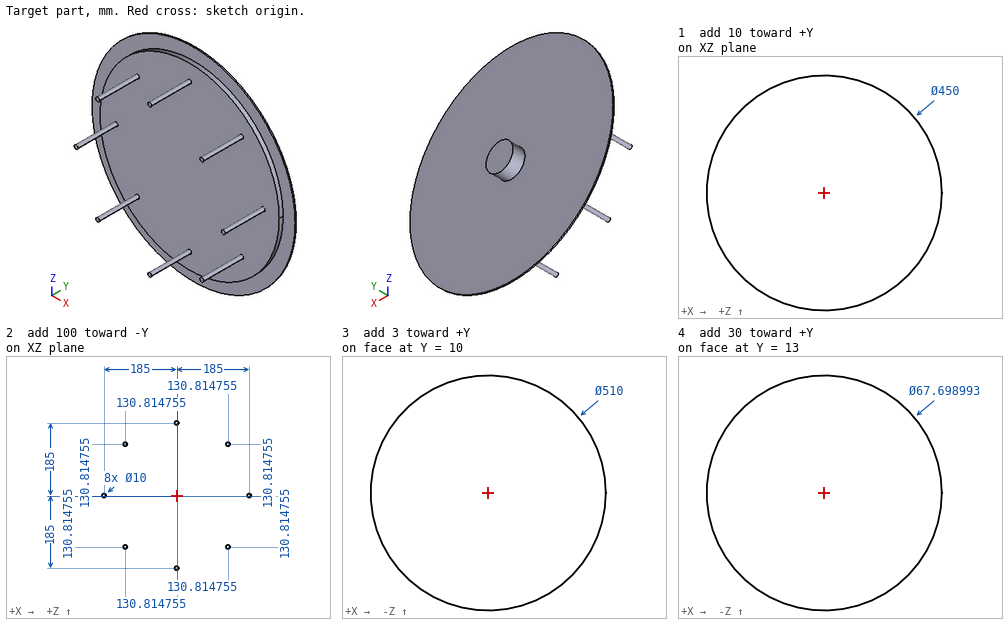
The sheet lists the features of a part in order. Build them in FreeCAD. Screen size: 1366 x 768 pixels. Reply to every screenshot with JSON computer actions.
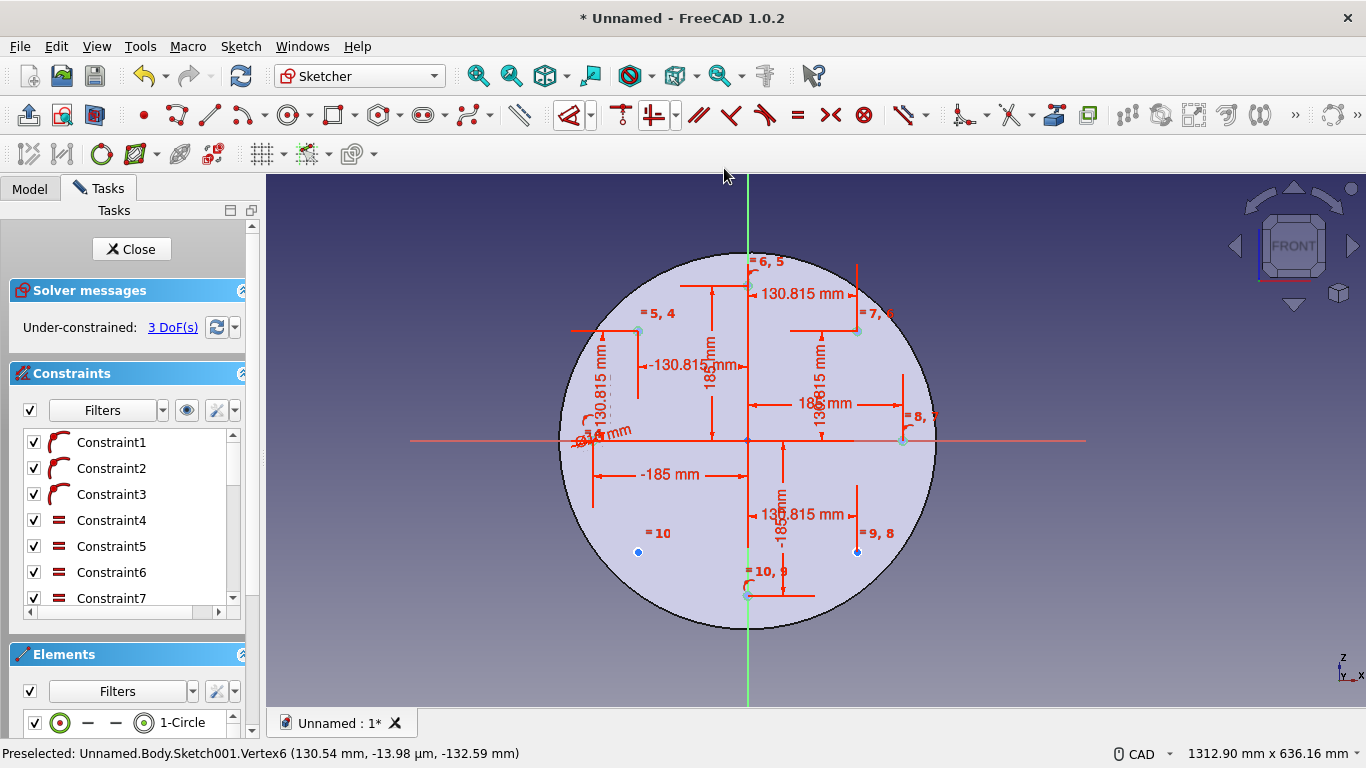
{"action": "left_click", "coordinate": [857, 552]}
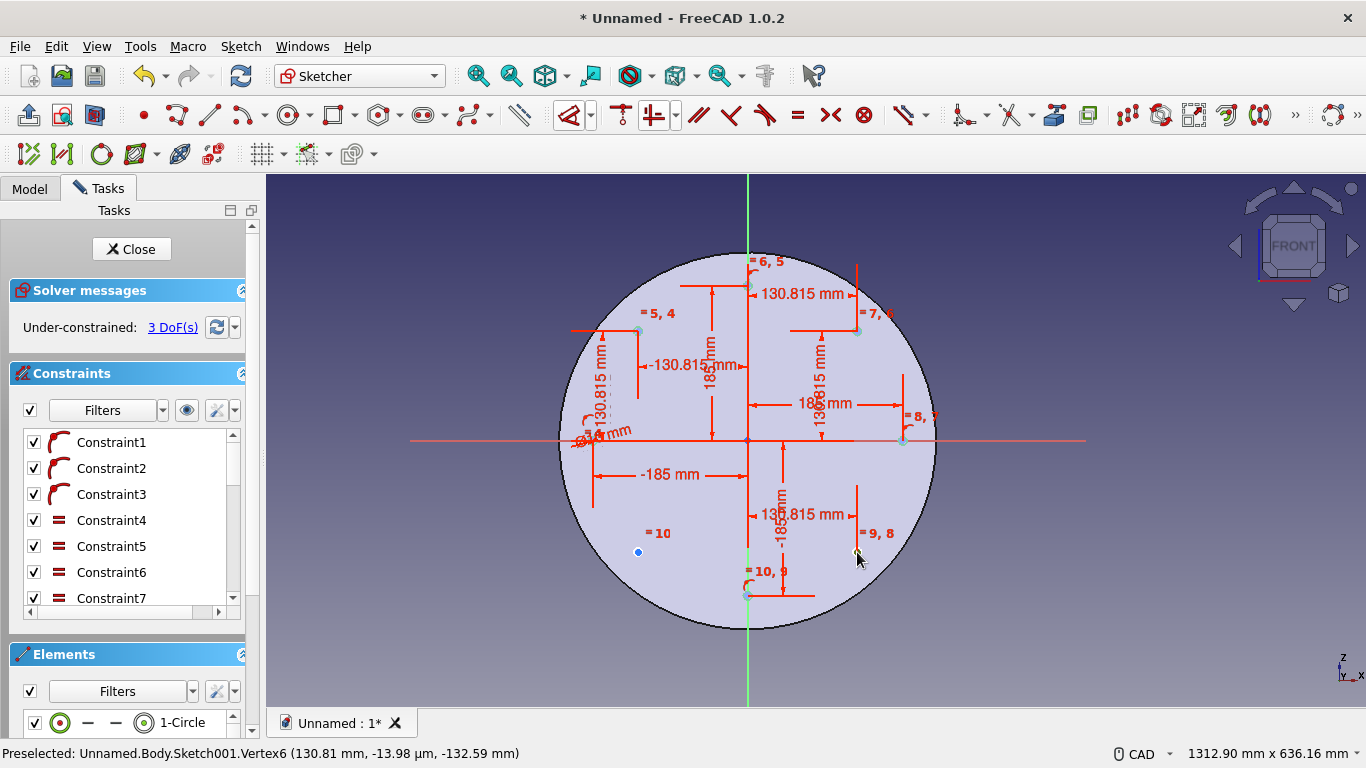
{"action": "left_click", "coordinate": [590, 116]}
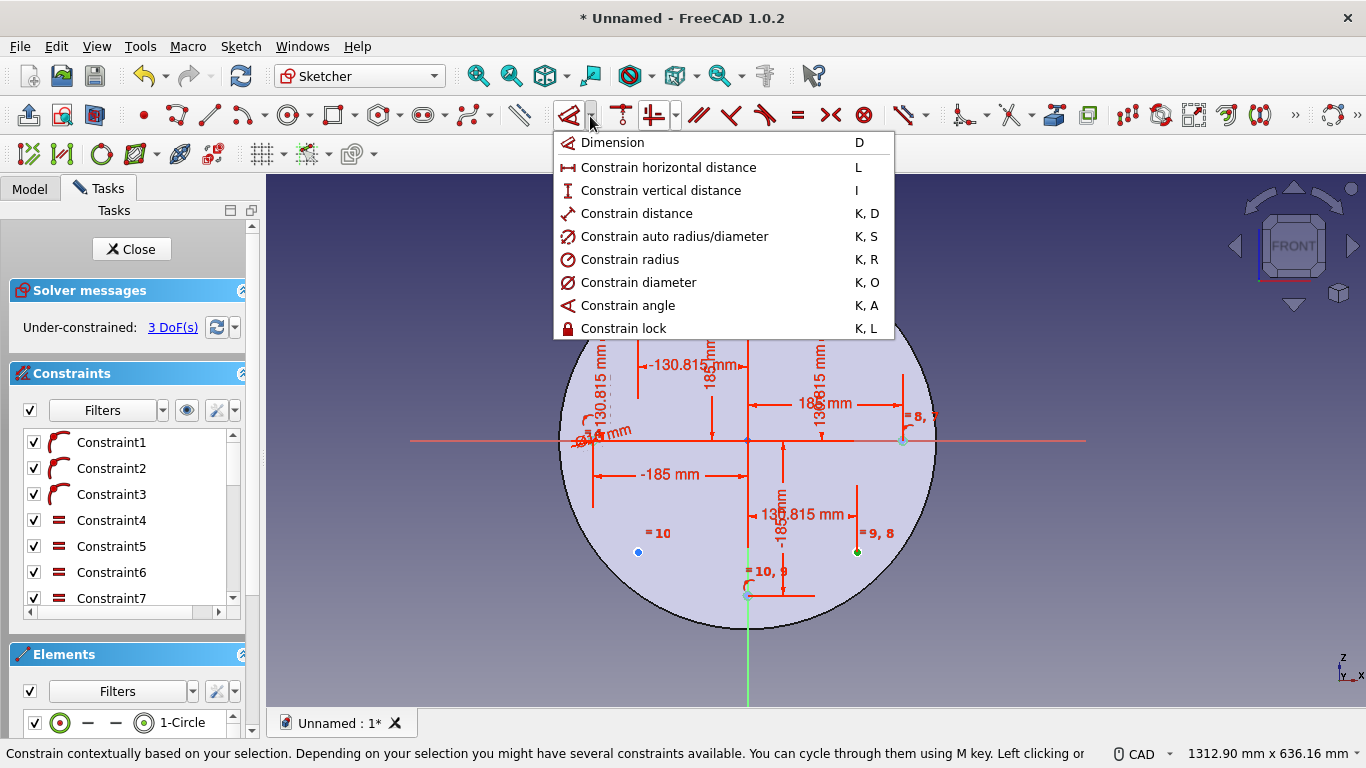
{"action": "left_click", "coordinate": [724, 190]}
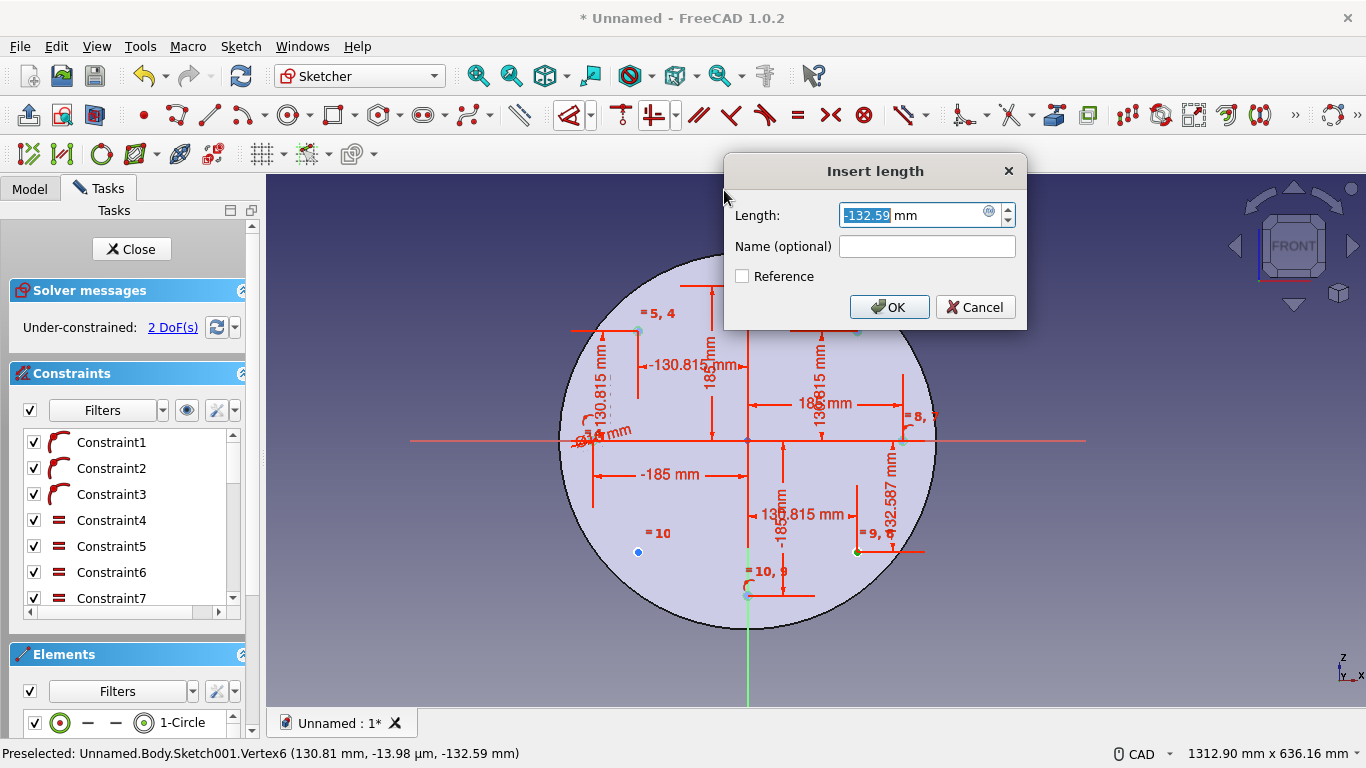
{"action": "type", "text": "-130.814755"}
{"action": "key", "text": "Return"}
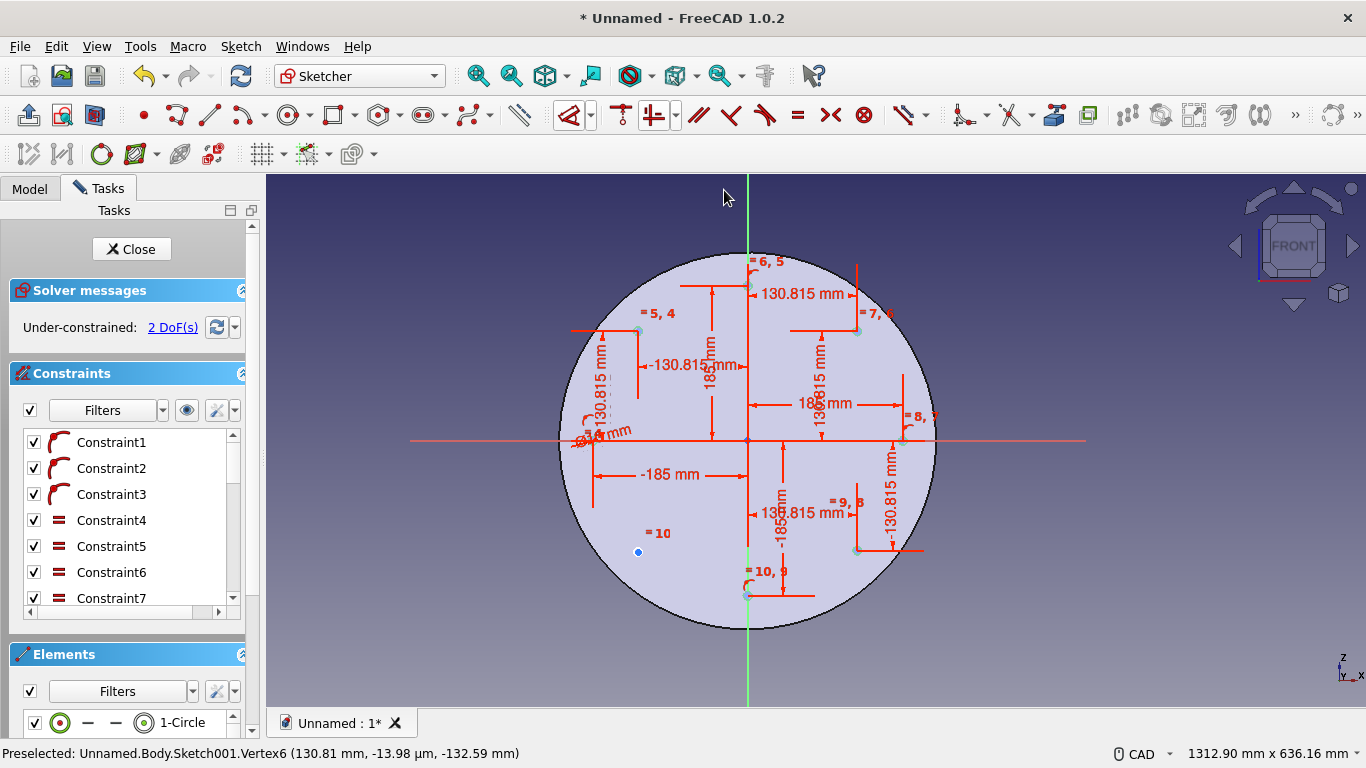
{"action": "left_click", "coordinate": [638, 552]}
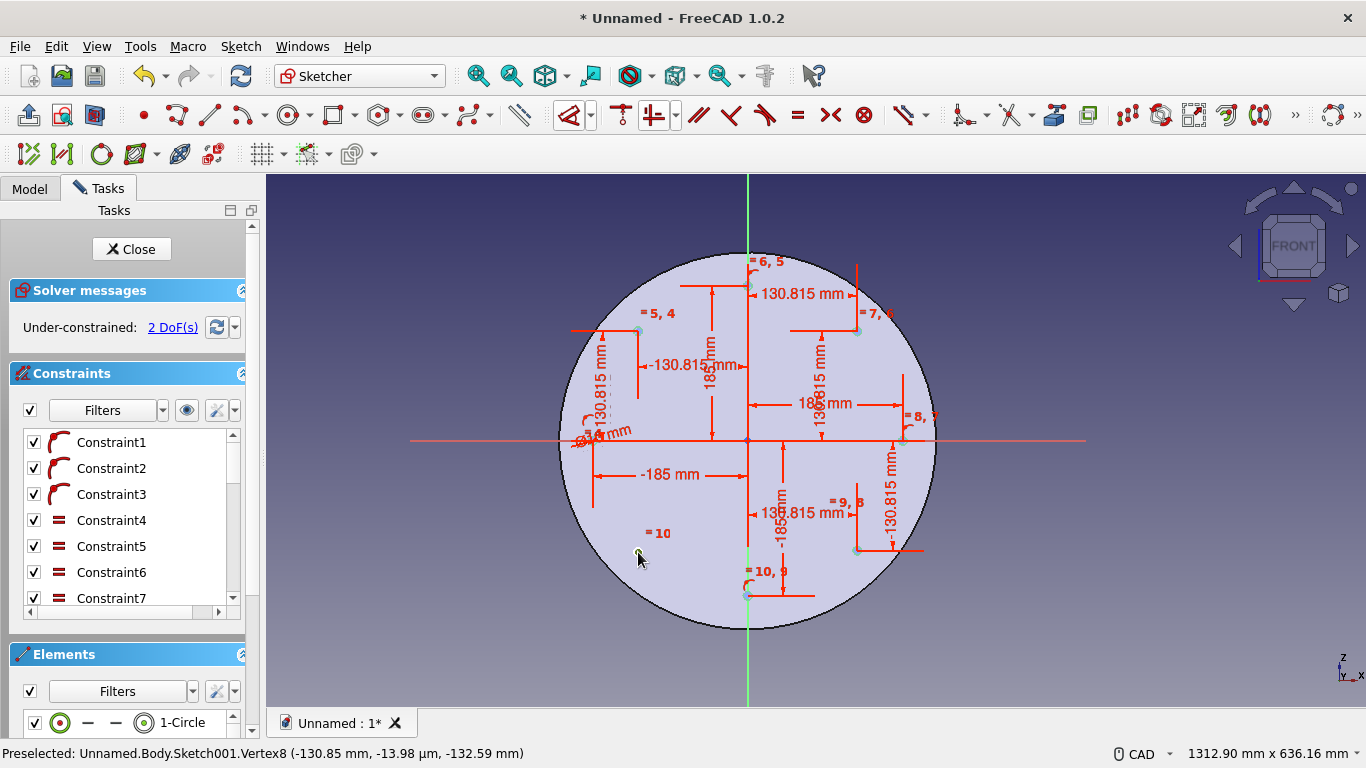
{"action": "left_click", "coordinate": [590, 116]}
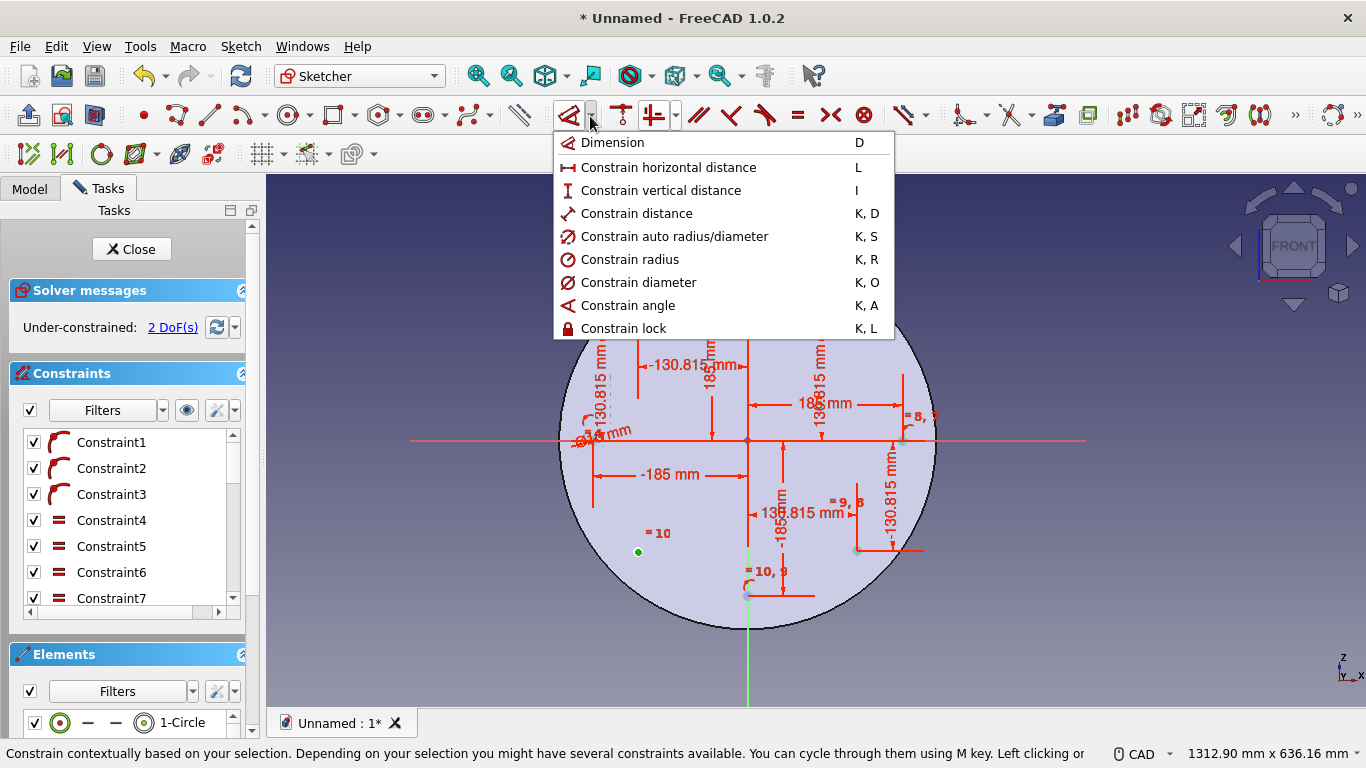
{"action": "left_click", "coordinate": [724, 168]}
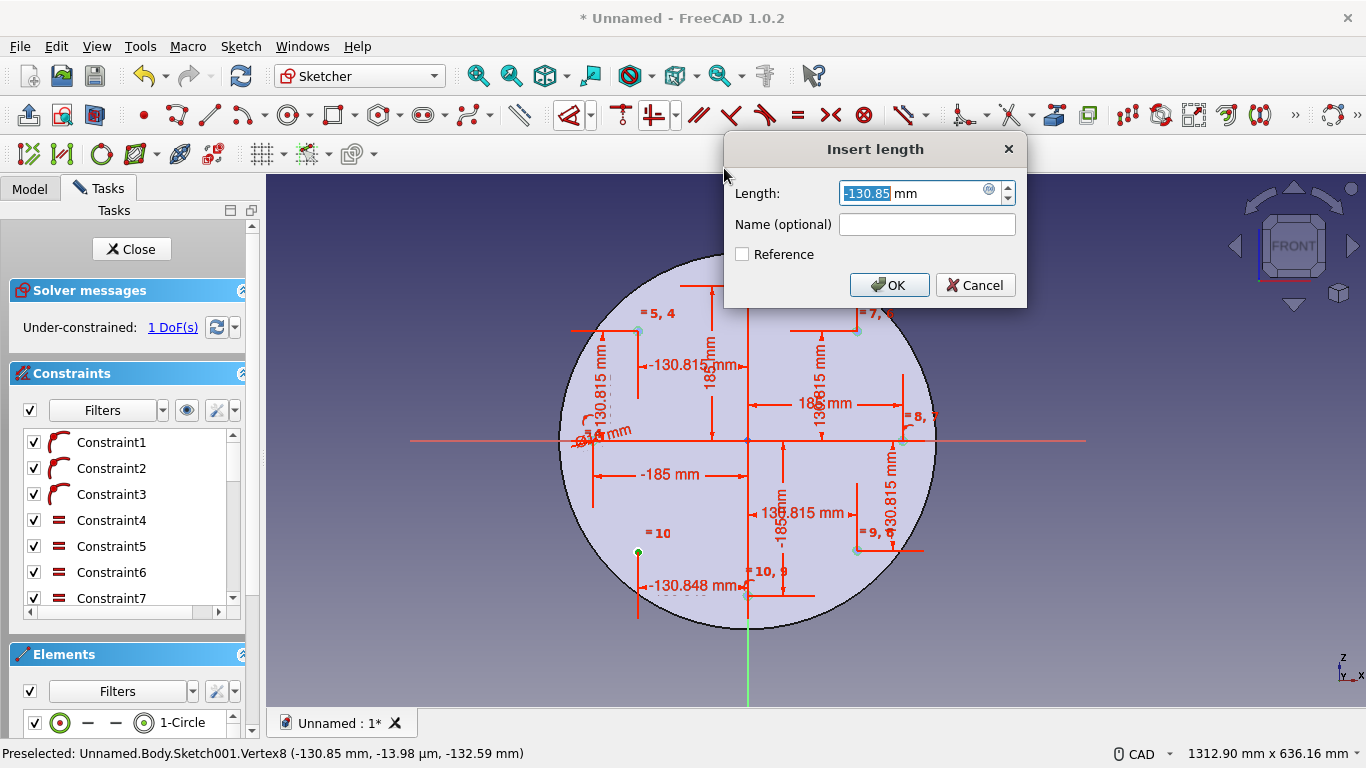
{"action": "type", "text": "-130.814755"}
{"action": "key", "text": "Return"}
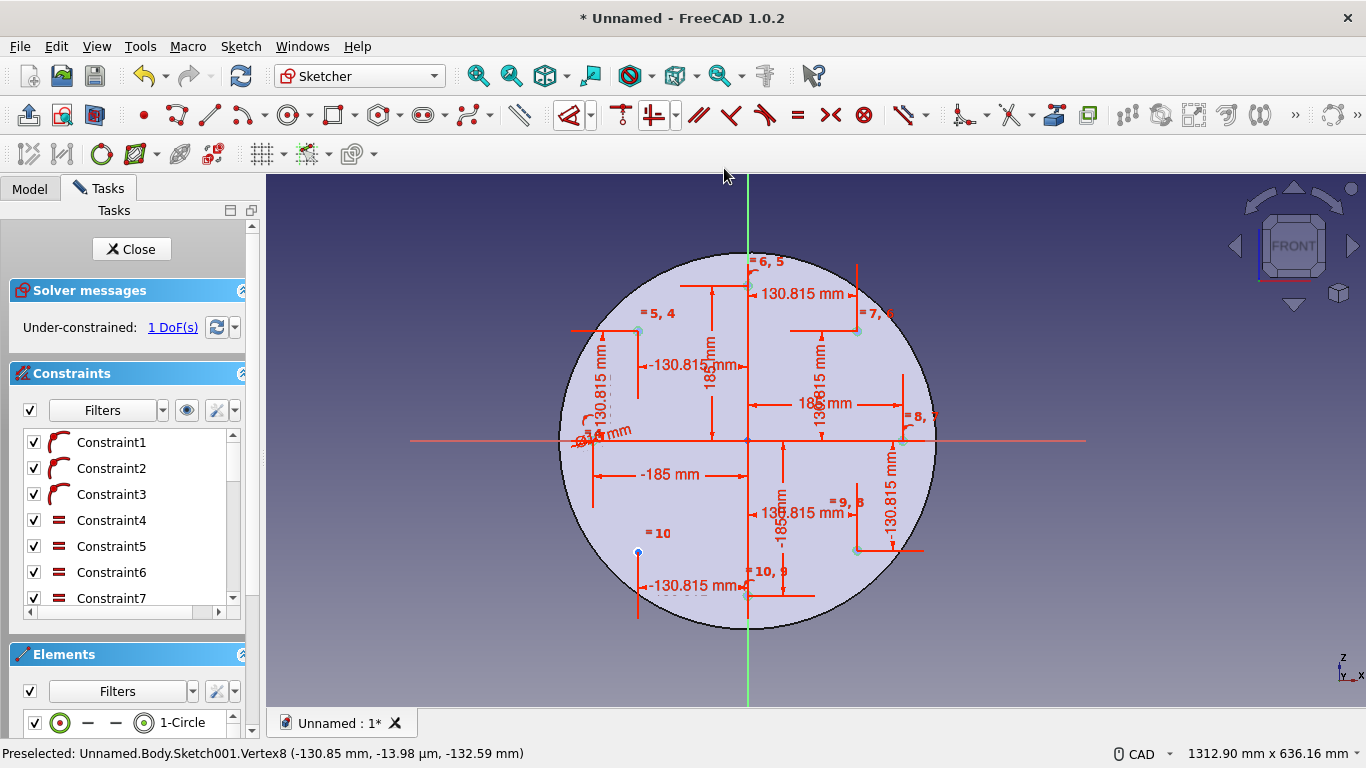
{"action": "left_click", "coordinate": [638, 552]}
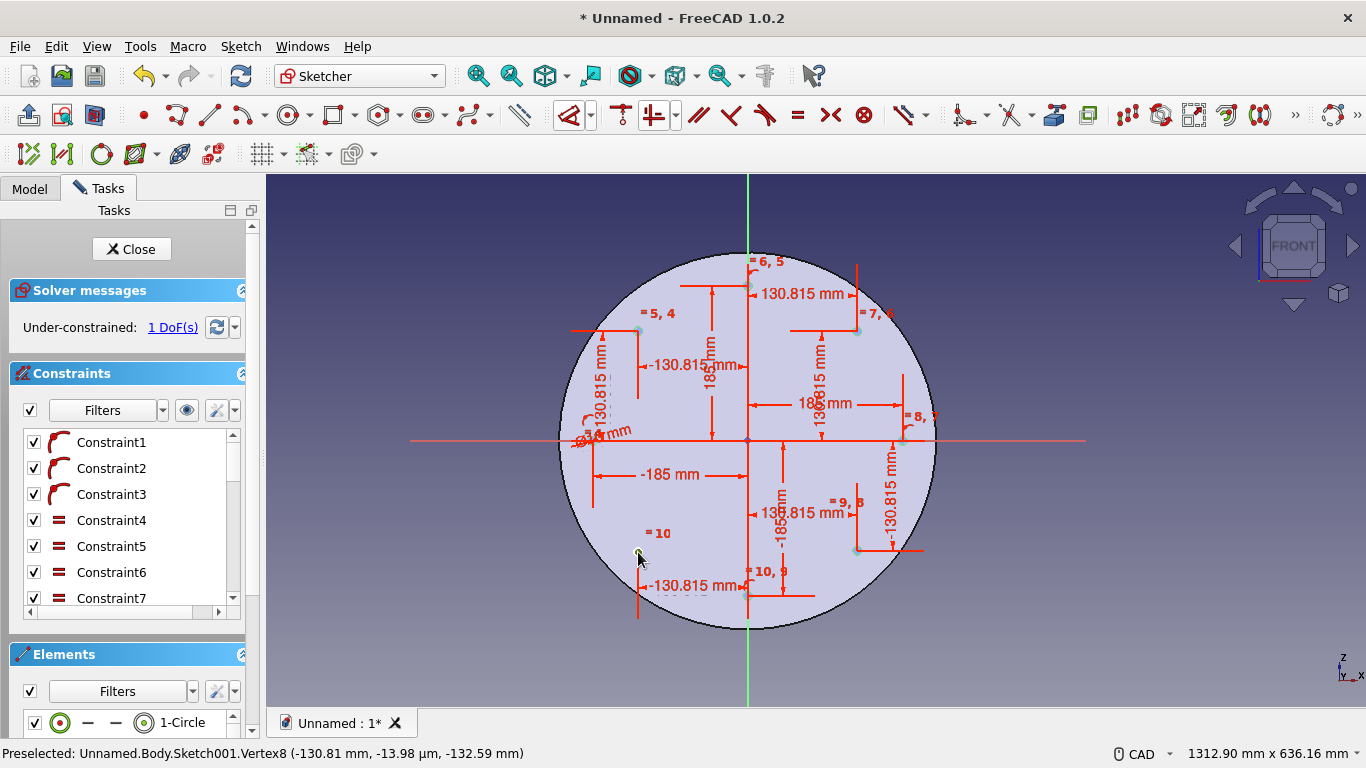
{"action": "left_click", "coordinate": [590, 116]}